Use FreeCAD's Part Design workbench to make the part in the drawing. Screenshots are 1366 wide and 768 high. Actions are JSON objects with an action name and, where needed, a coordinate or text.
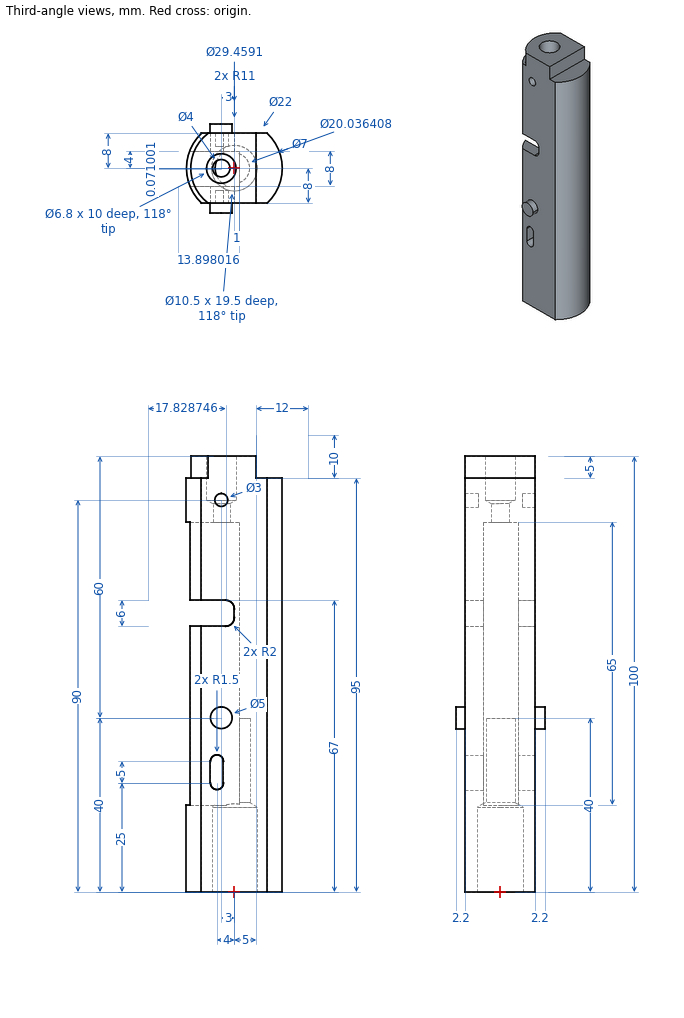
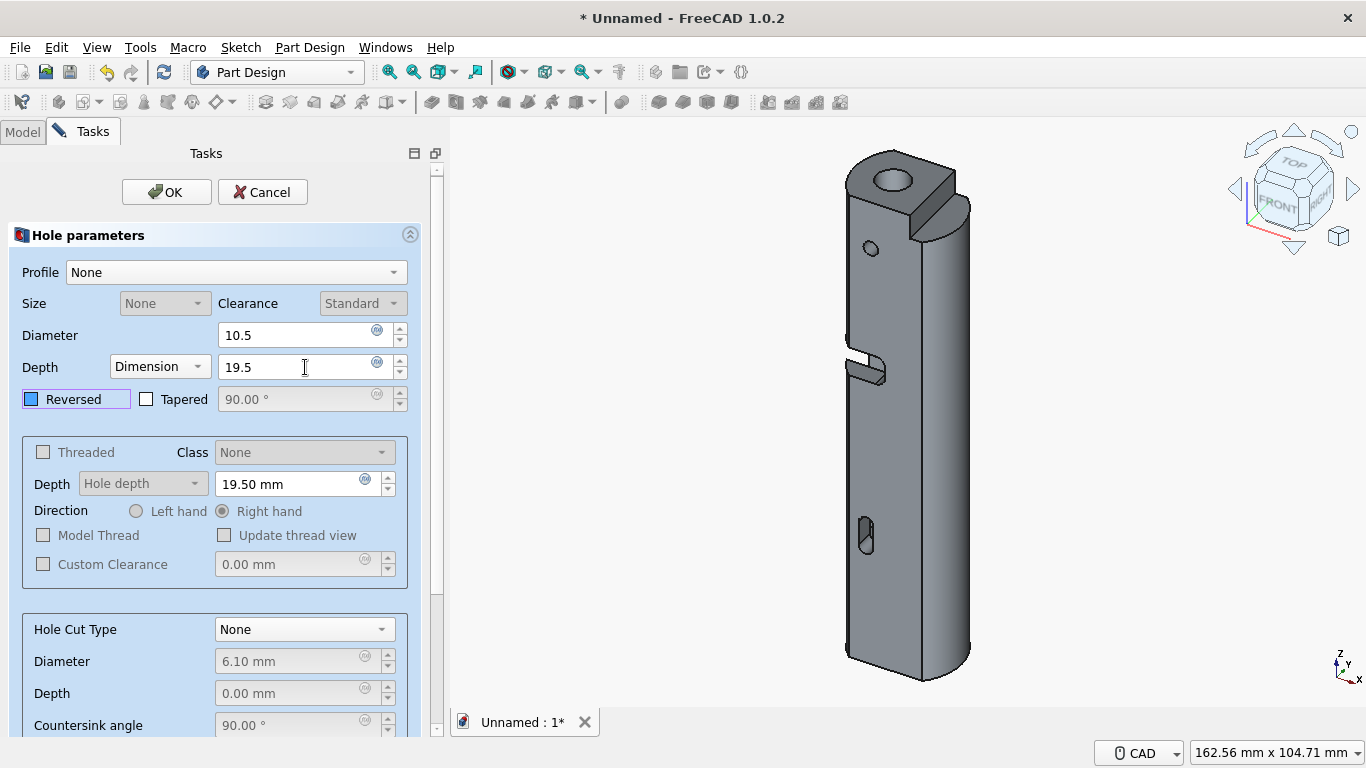
{"action": "left_click", "coordinate": [30, 399]}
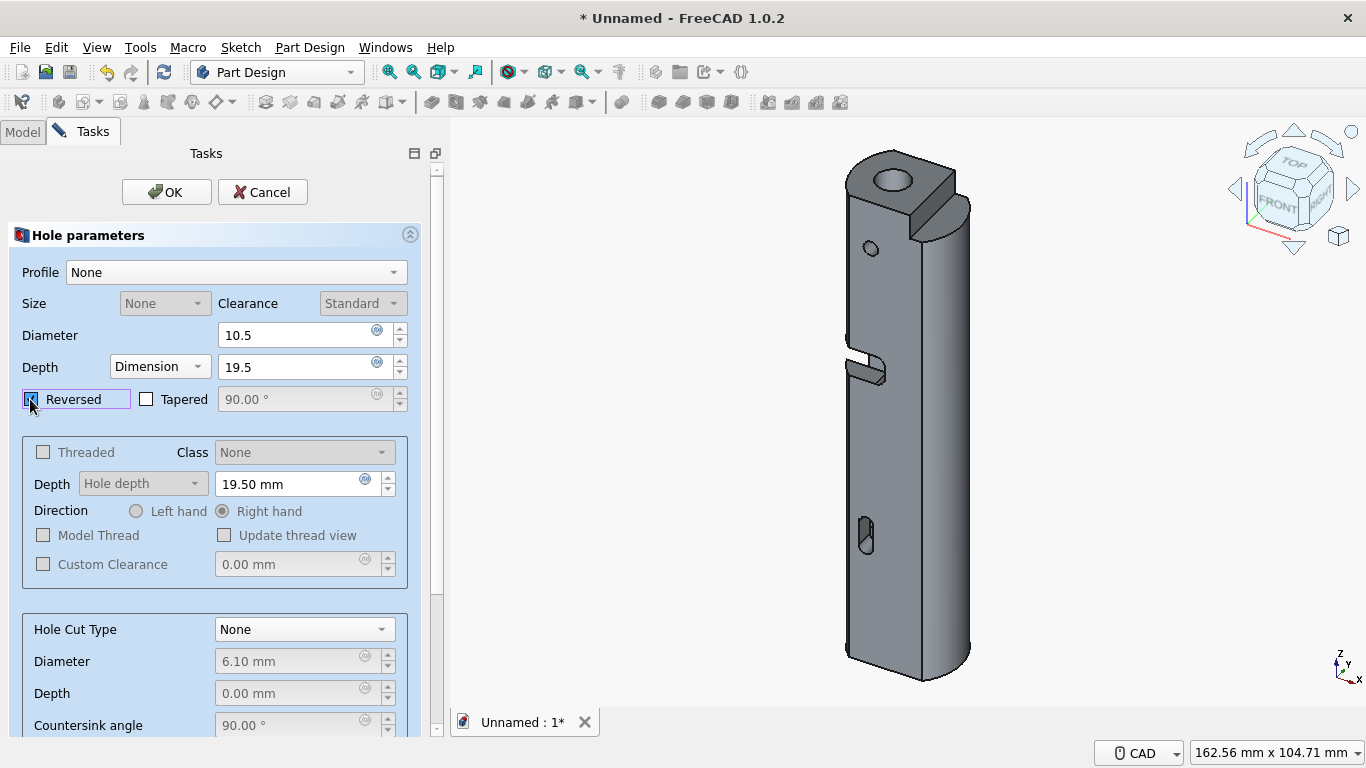
{"action": "left_click", "coordinate": [167, 192]}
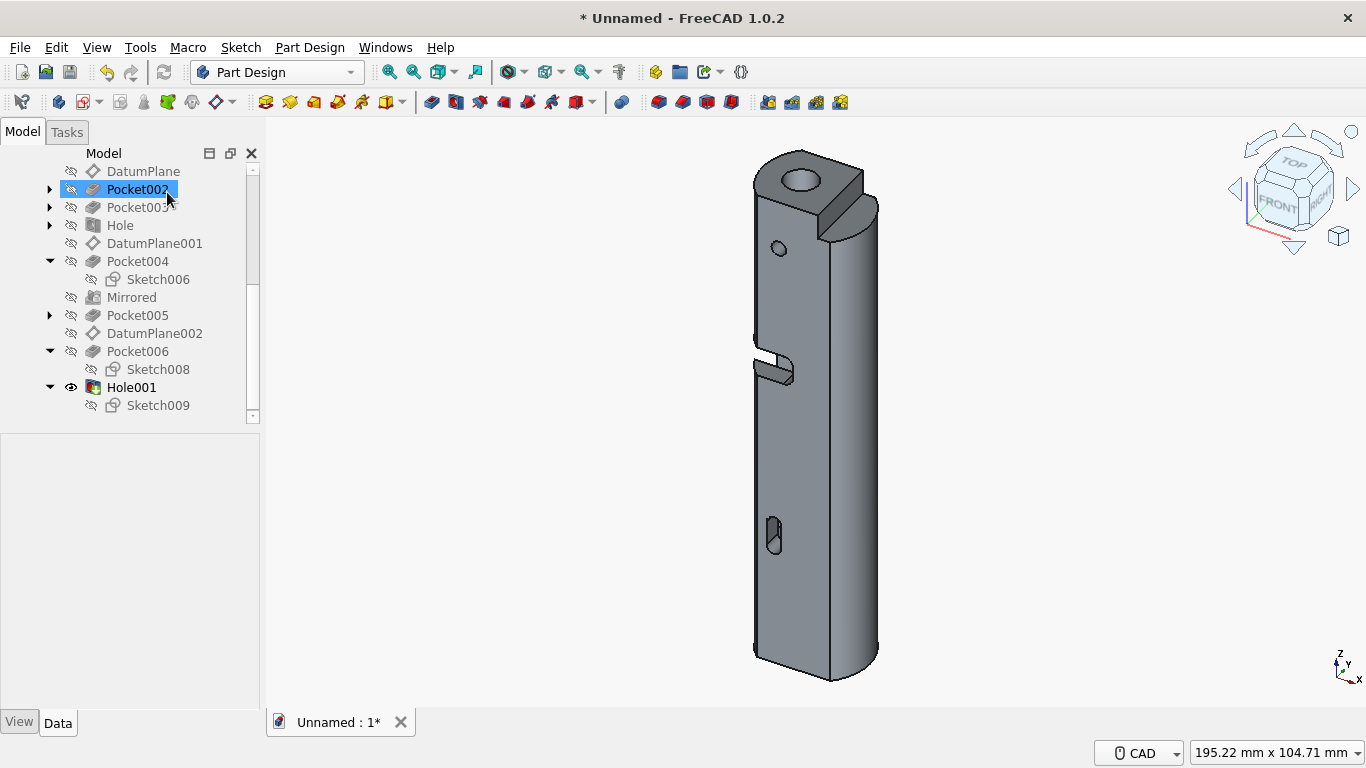
{"action": "left_click", "coordinate": [793, 305]}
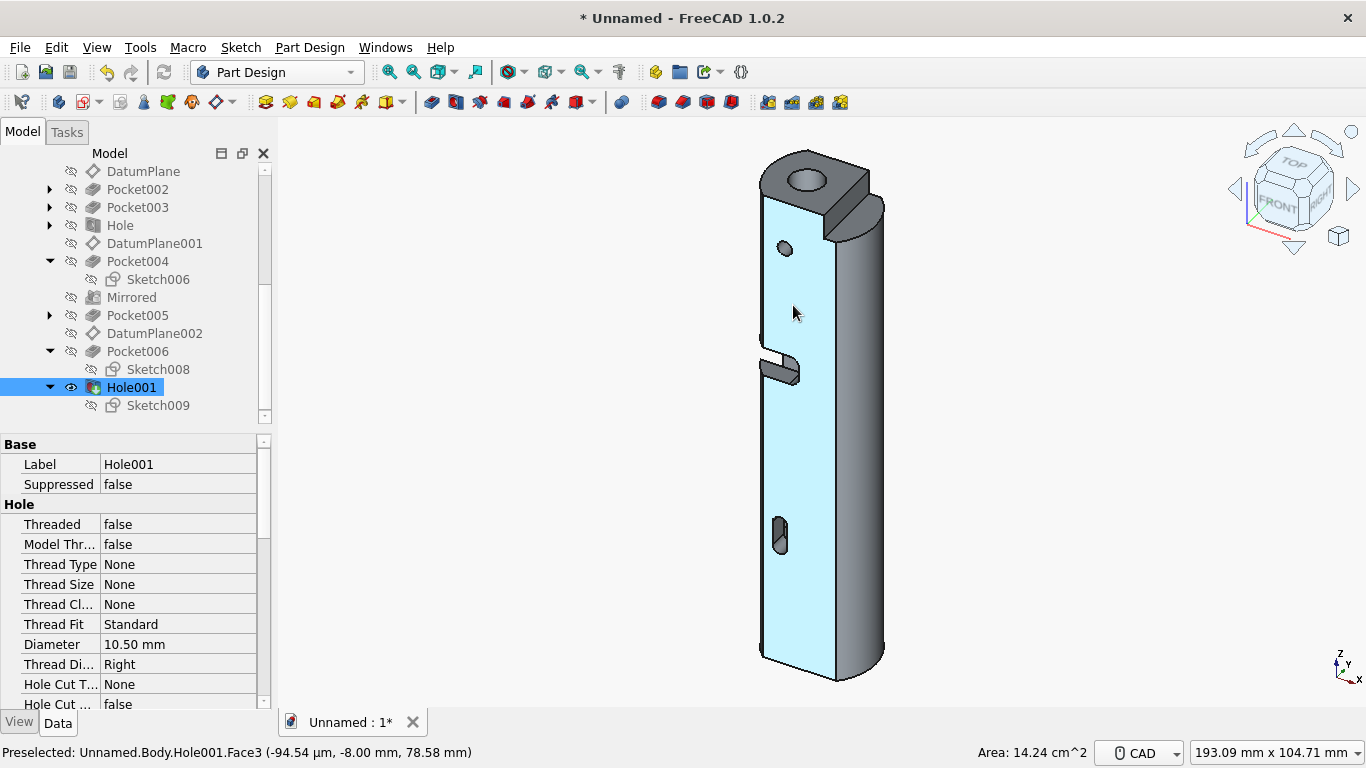
{"action": "left_click", "coordinate": [84, 102]}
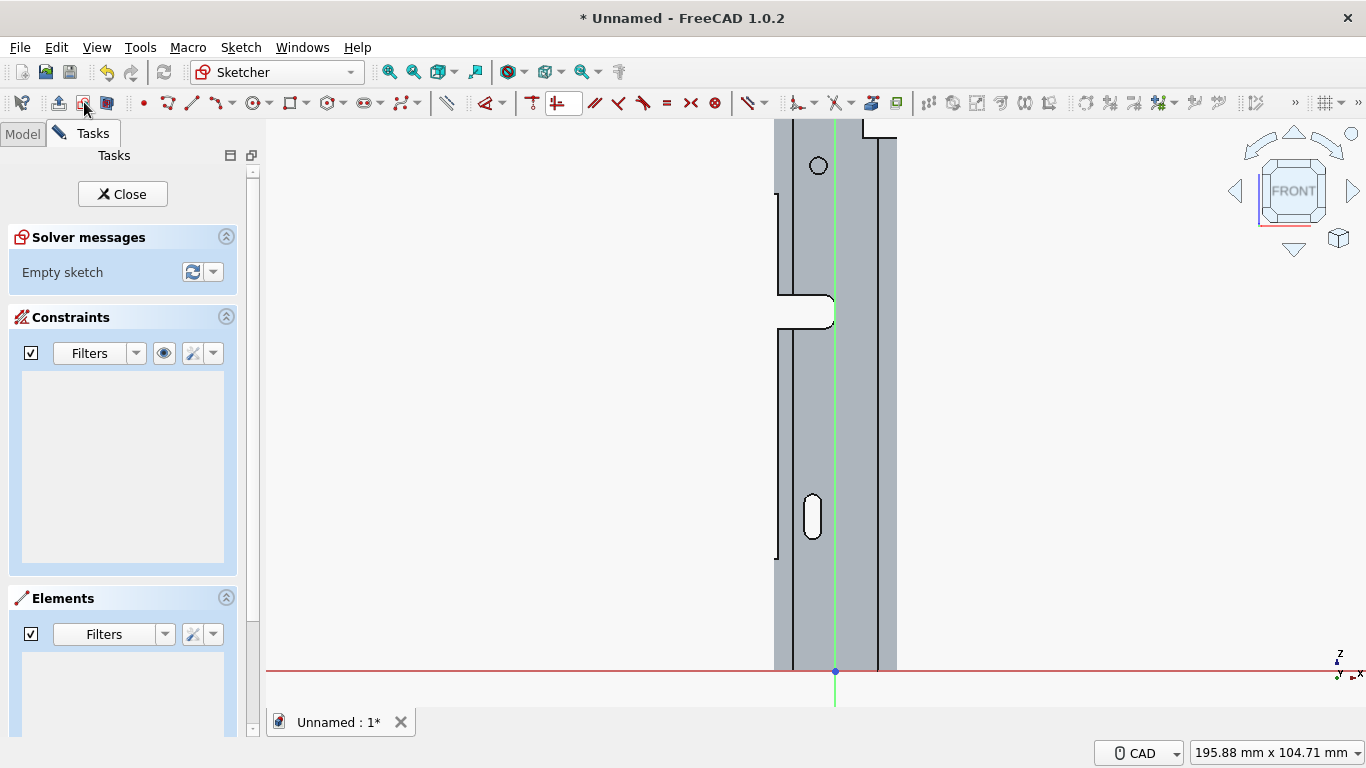
{"action": "scroll", "coordinate": [824, 449], "scroll_direction": "up", "scroll_amount": 13}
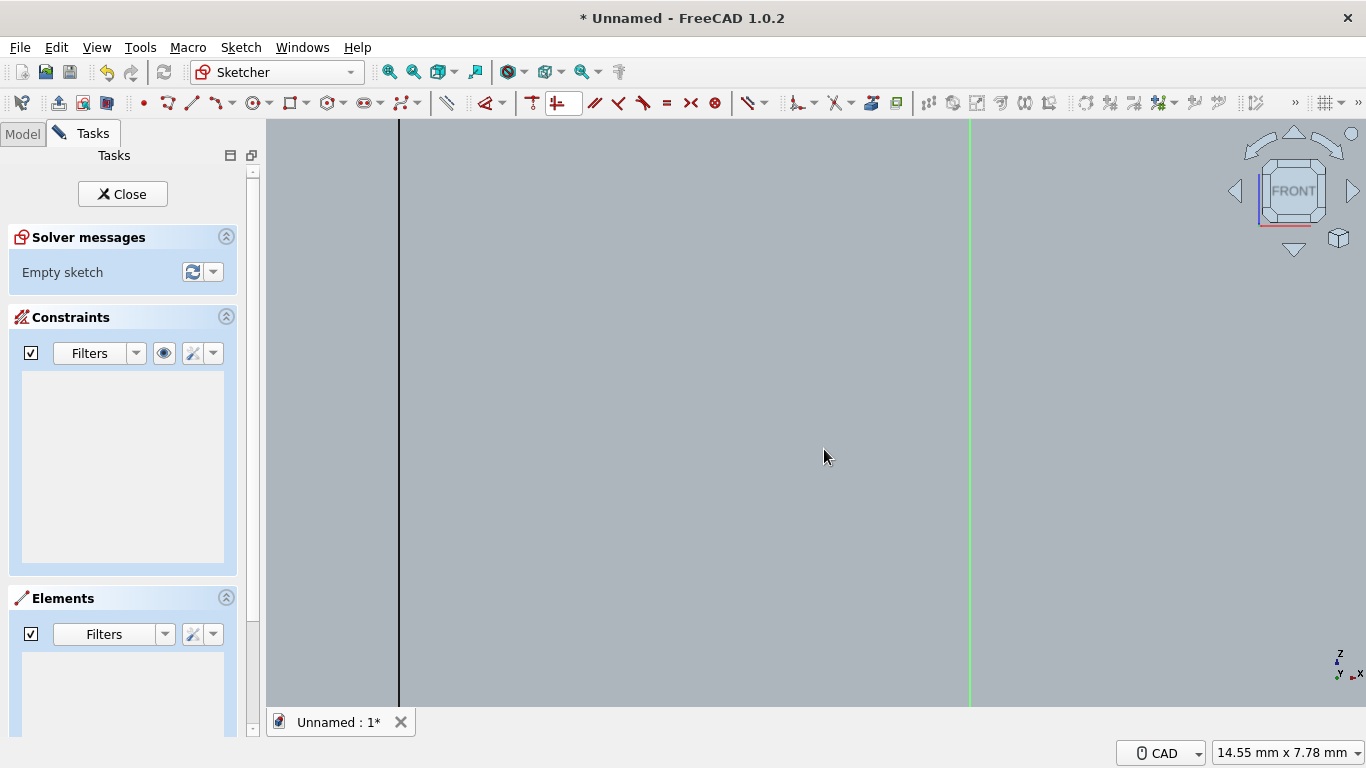
{"action": "key", "text": "g c"}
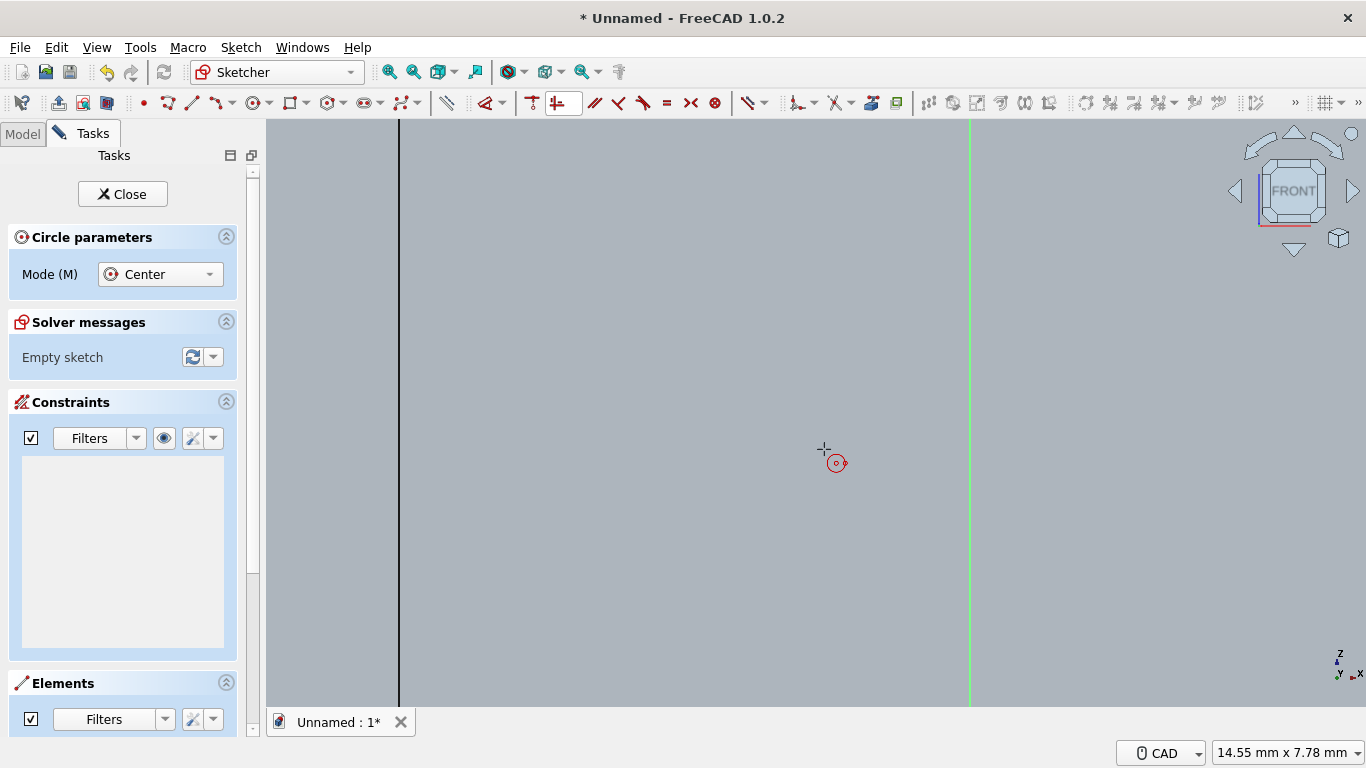
{"action": "left_click", "coordinate": [743, 410]}
{"action": "mouse_move", "coordinate": [877, 276]}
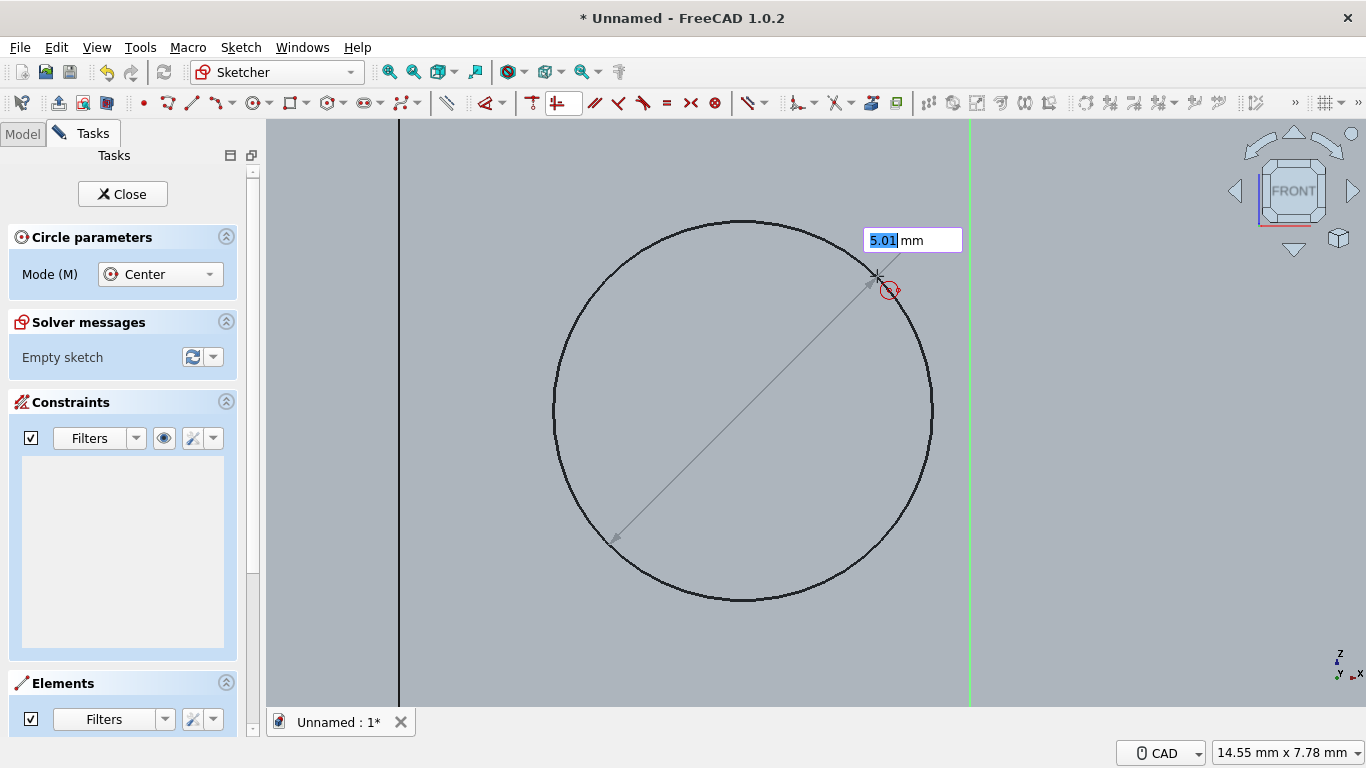
{"action": "type", "text": "5"}
{"action": "key", "text": "Return"}
{"action": "key", "text": "Escape"}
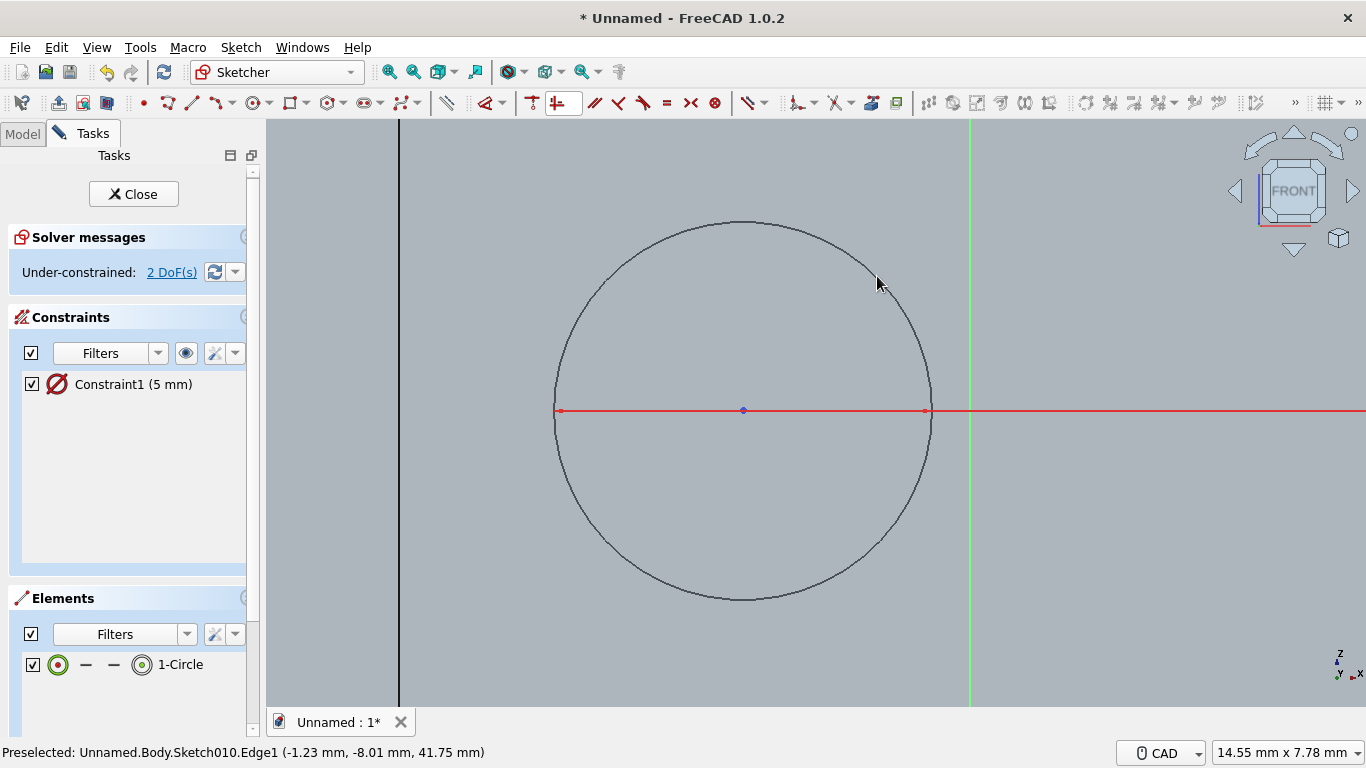
{"action": "key", "text": "d"}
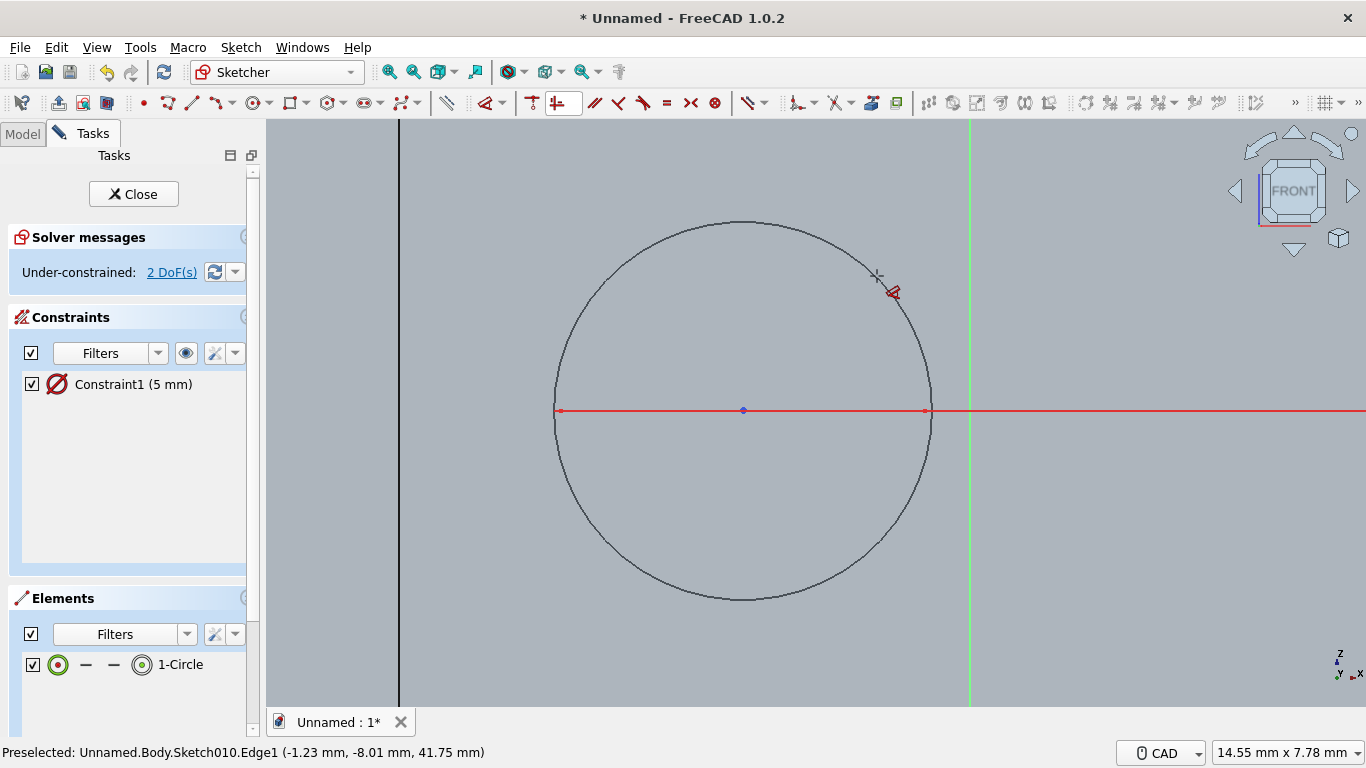
{"action": "left_click", "coordinate": [743, 411]}
{"action": "left_click", "coordinate": [856, 377]}